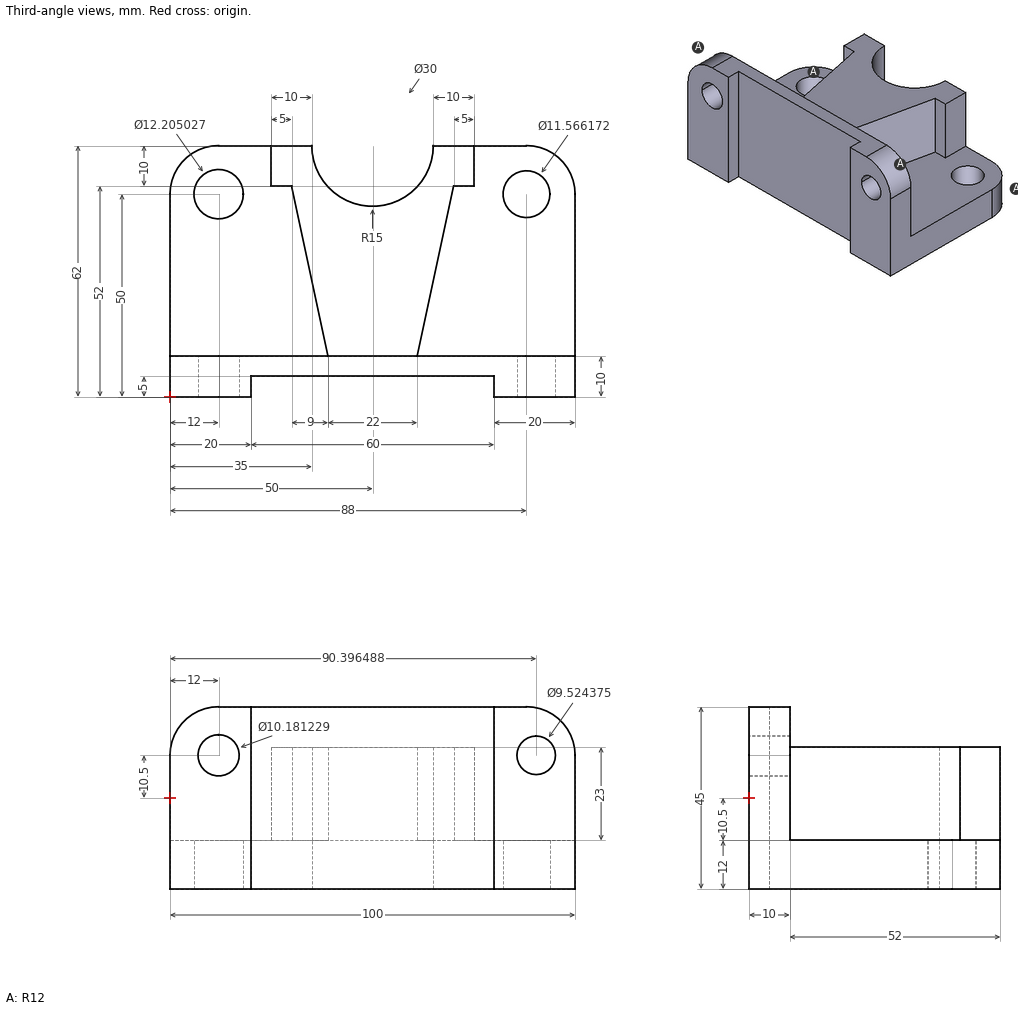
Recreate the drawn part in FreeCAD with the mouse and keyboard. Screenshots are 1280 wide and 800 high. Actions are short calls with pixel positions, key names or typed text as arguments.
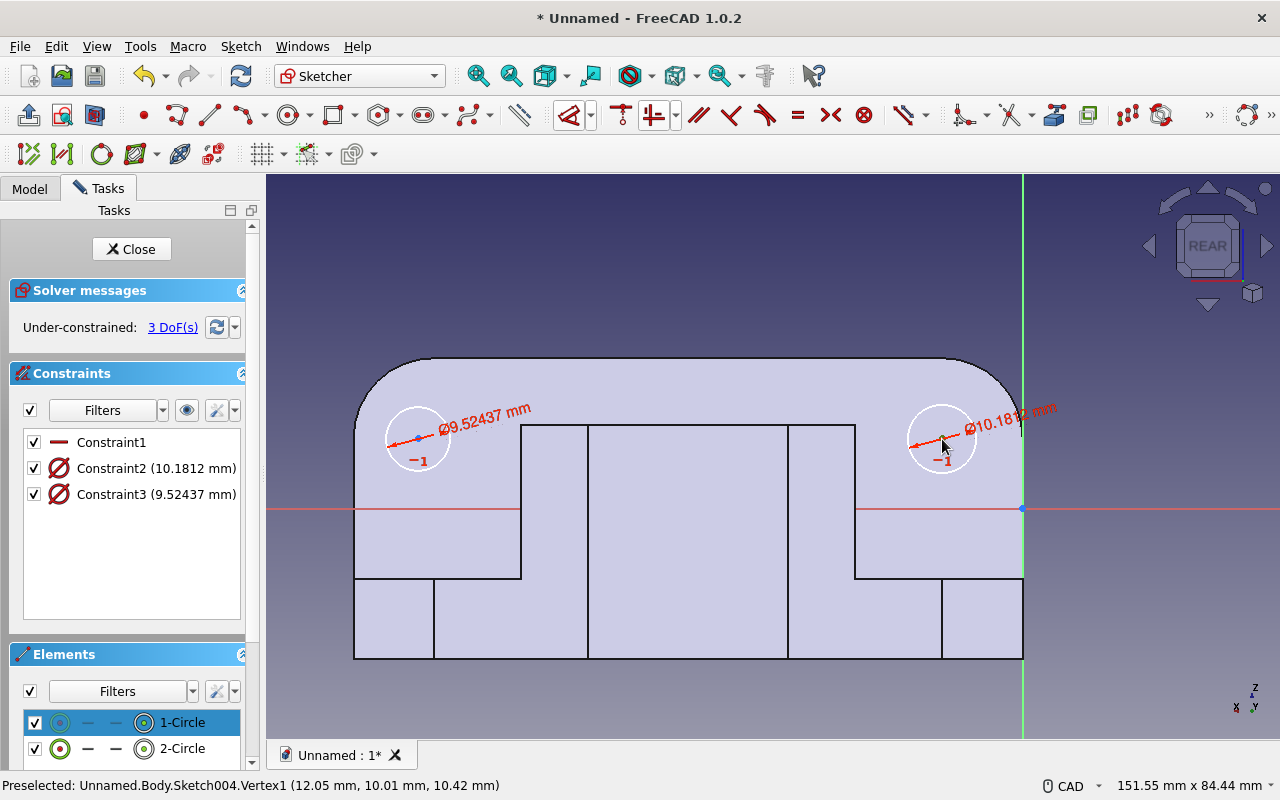
key(l)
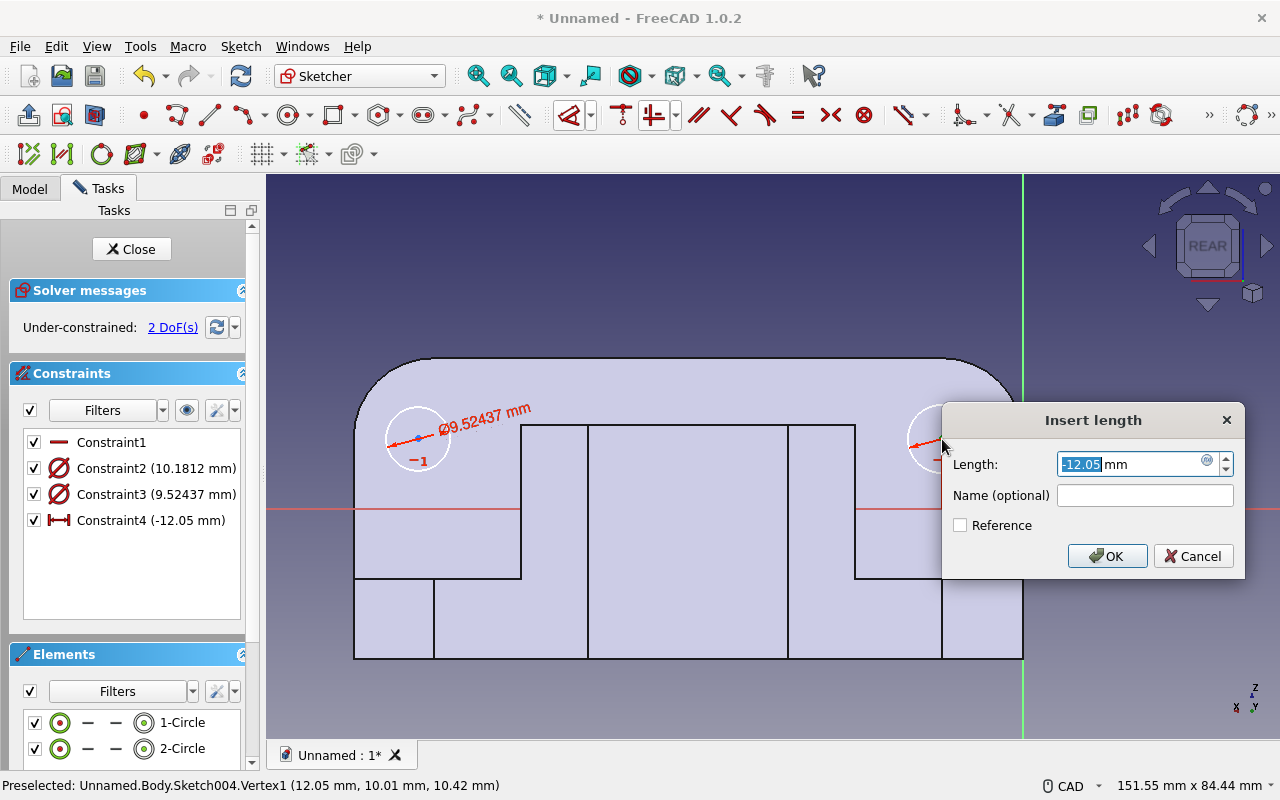
text(-12)
key(Return)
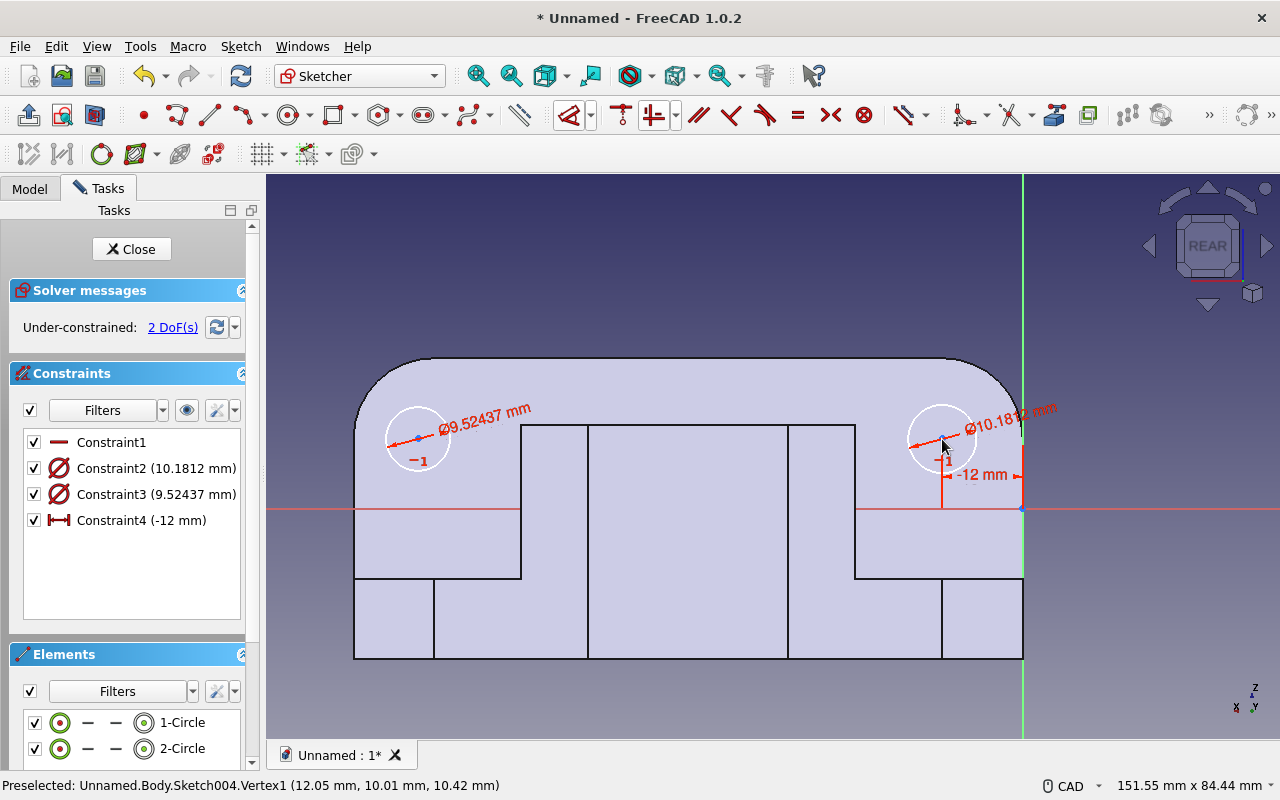
click(942, 439)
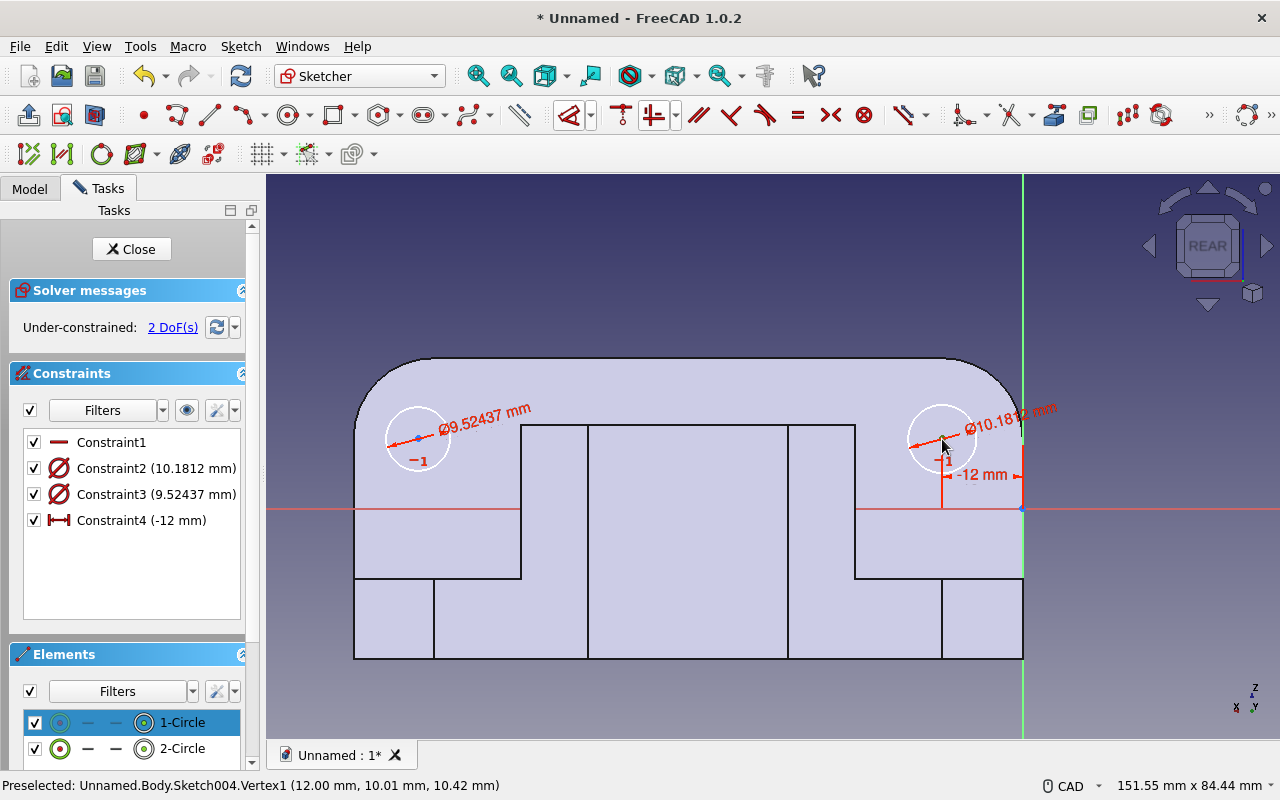
key(i)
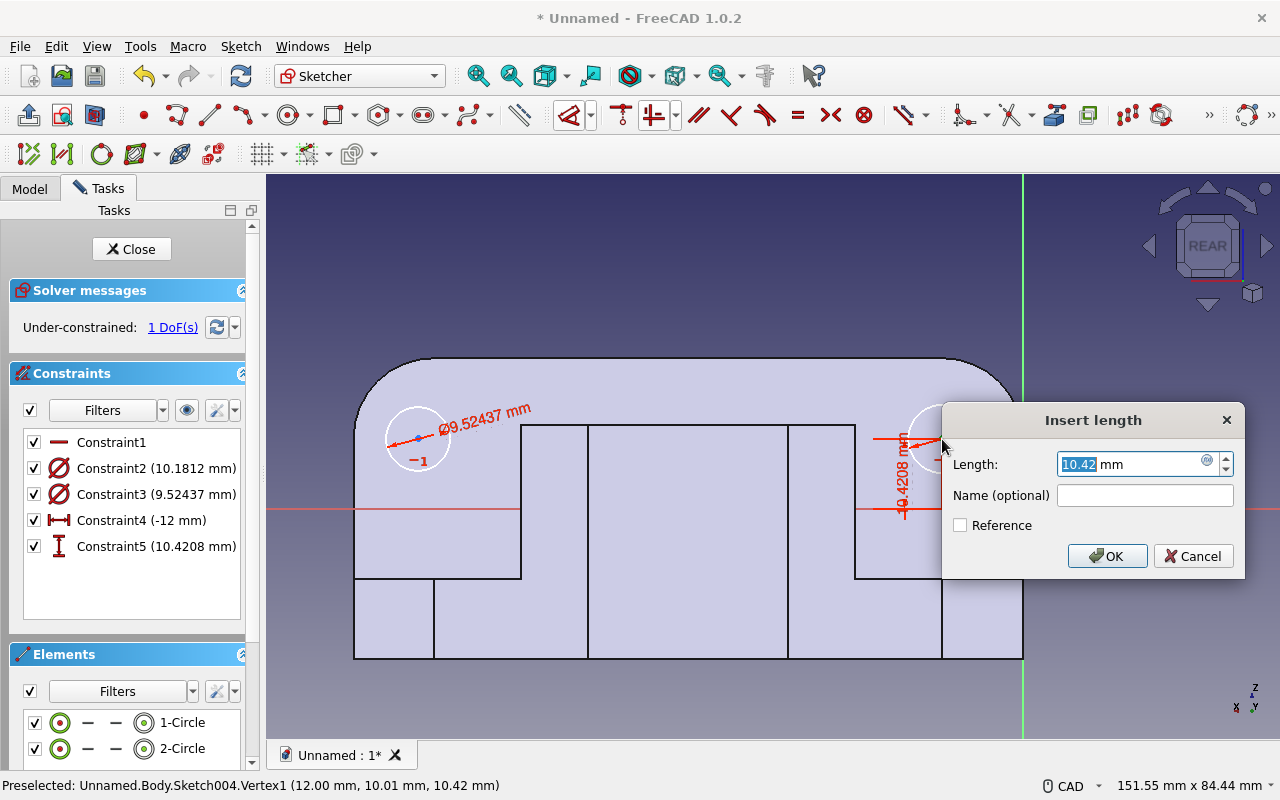
text(10.5)
key(Return)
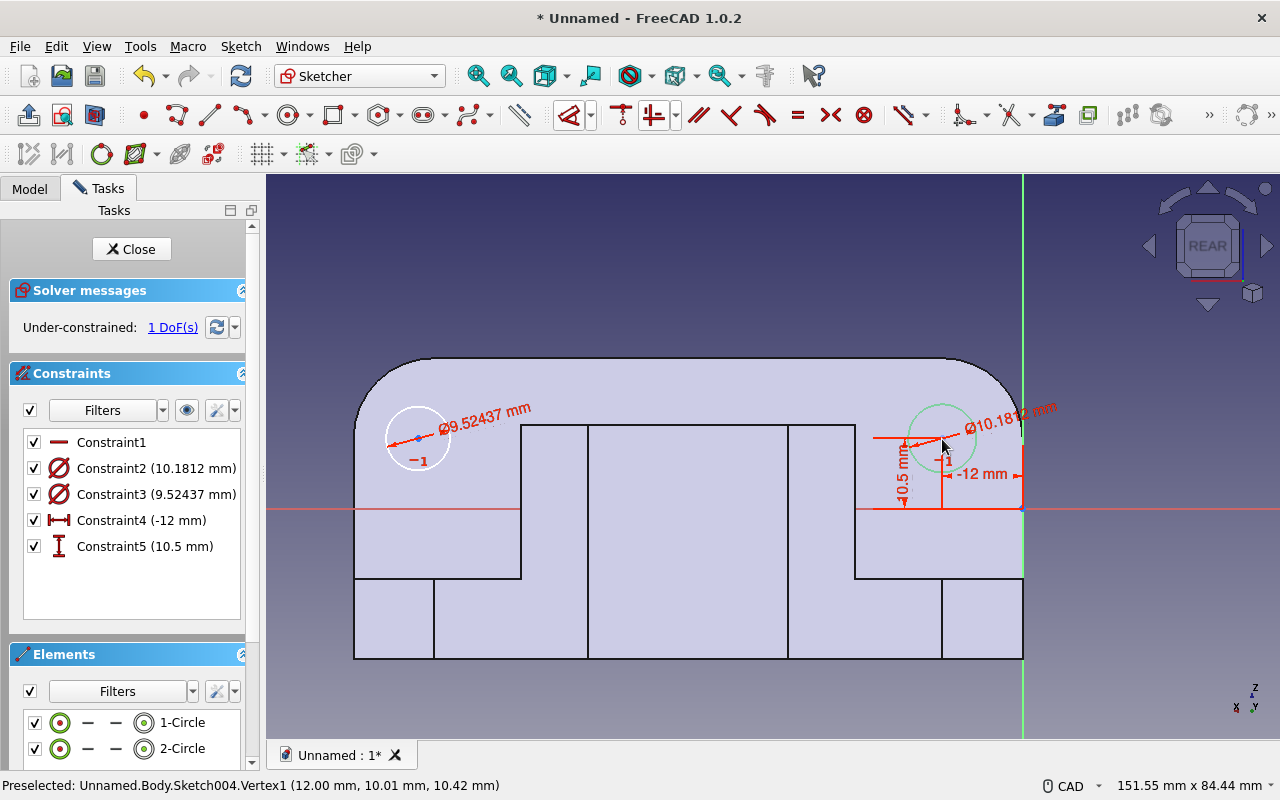
click(418, 438)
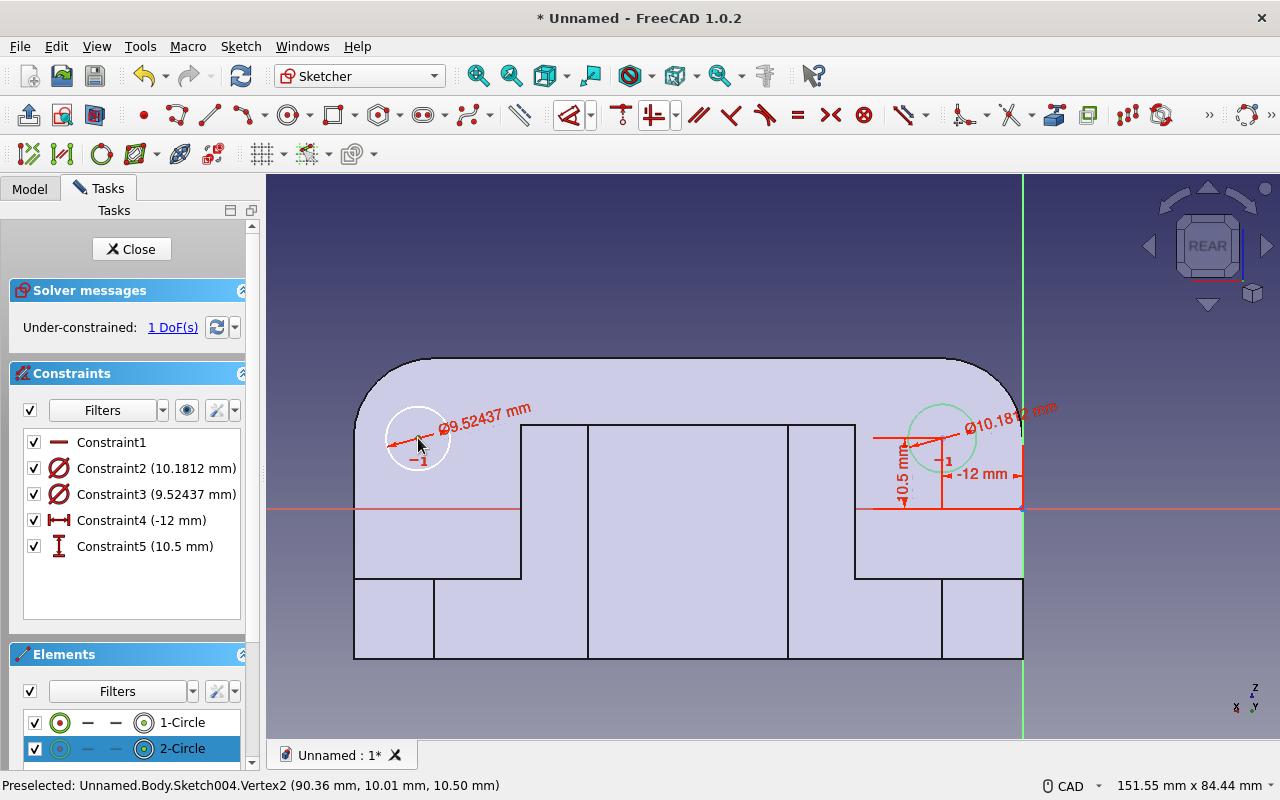
key(l)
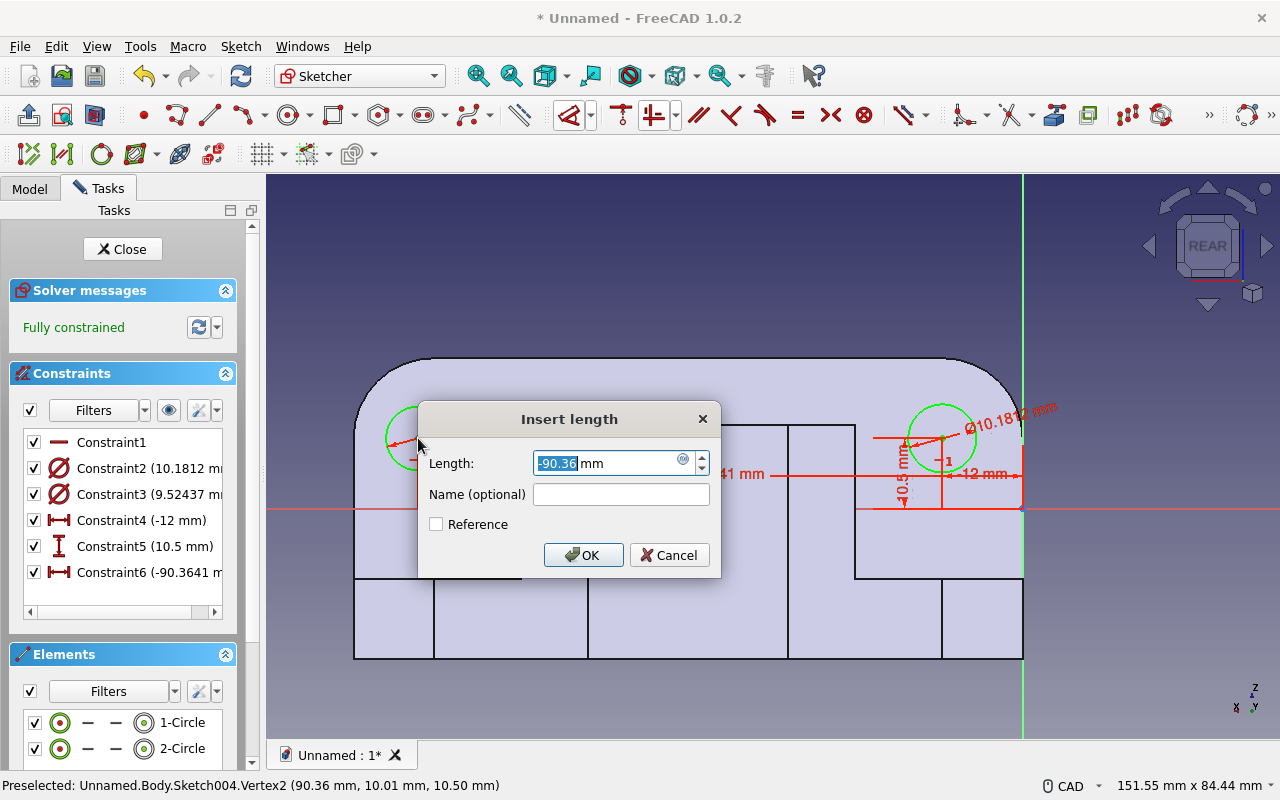
text(-90.396488)
key(Return)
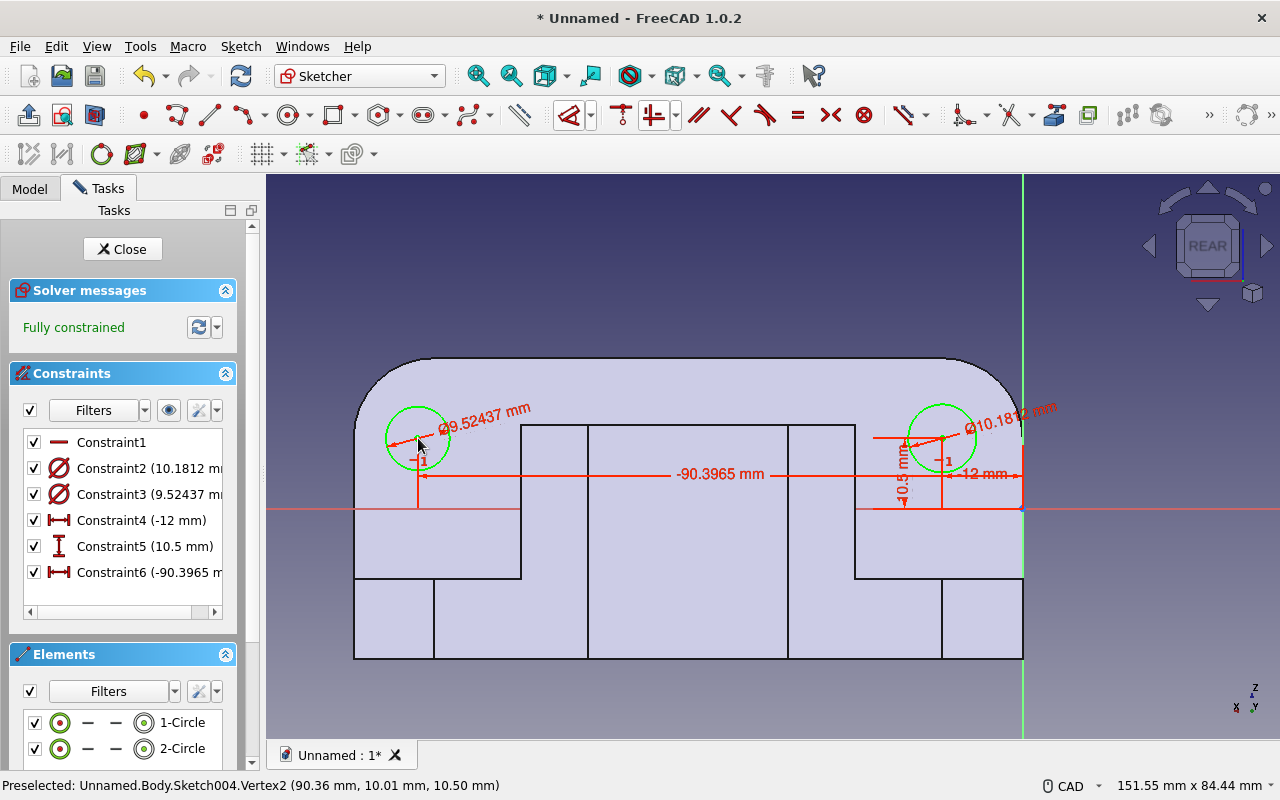
click(123, 249)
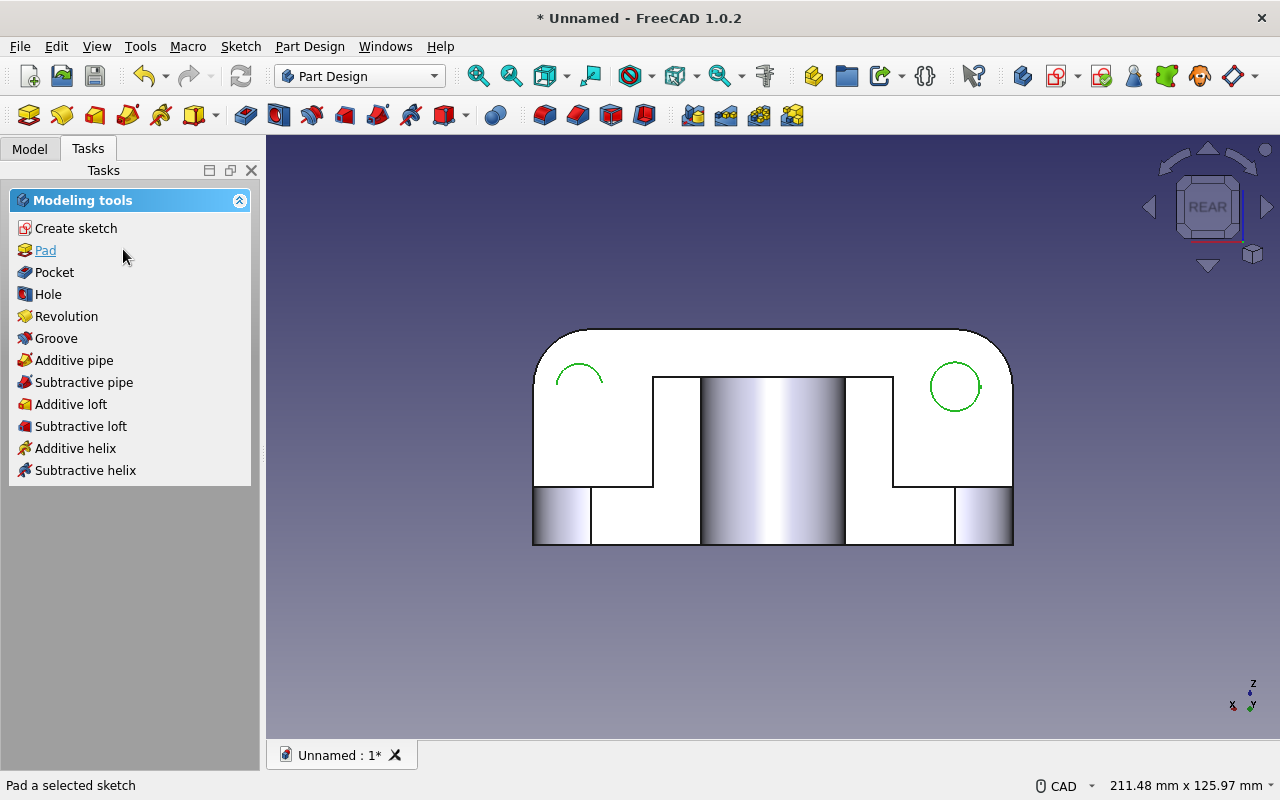
click(246, 116)